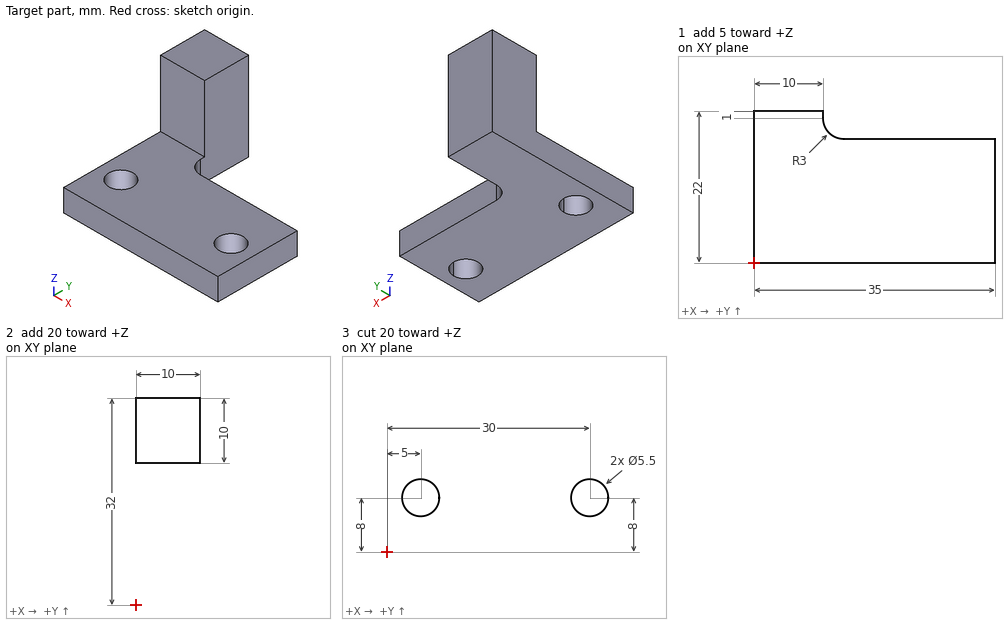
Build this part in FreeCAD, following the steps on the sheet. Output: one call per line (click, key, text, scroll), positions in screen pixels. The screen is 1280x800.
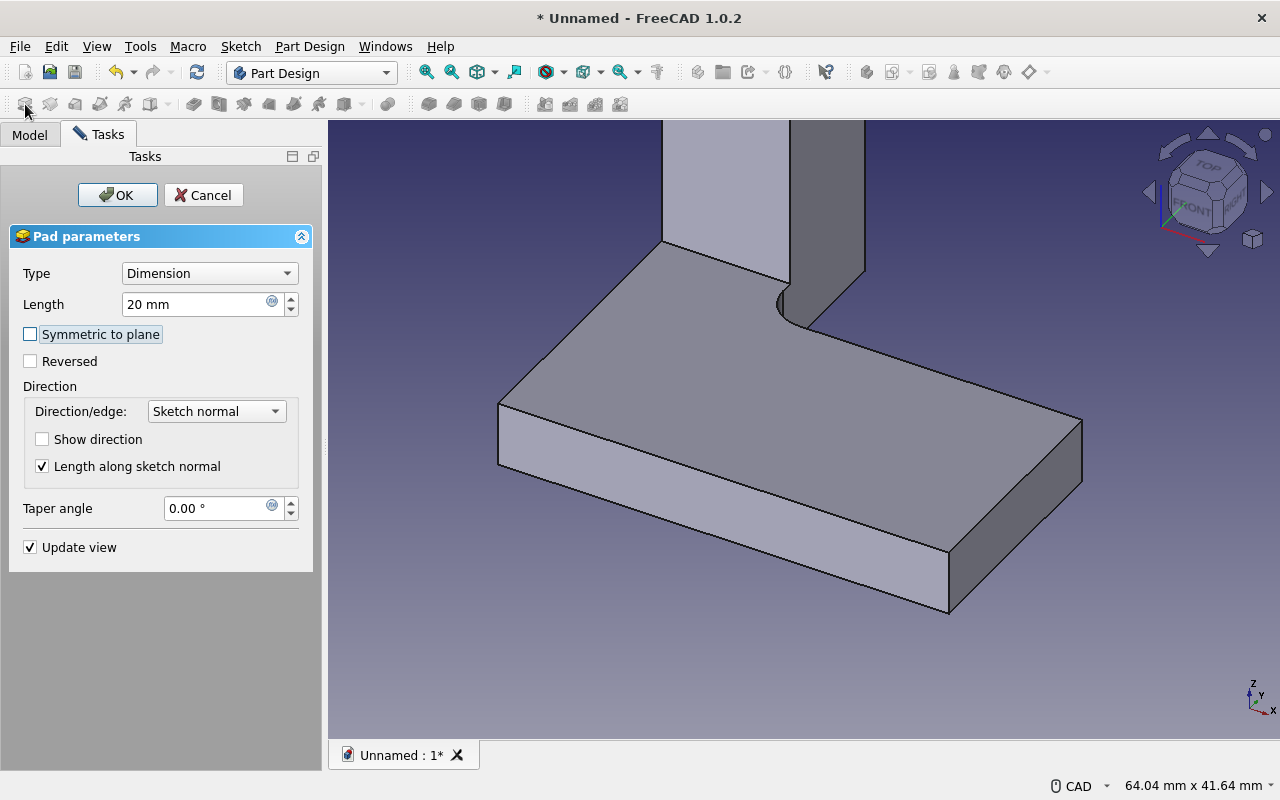
click(118, 195)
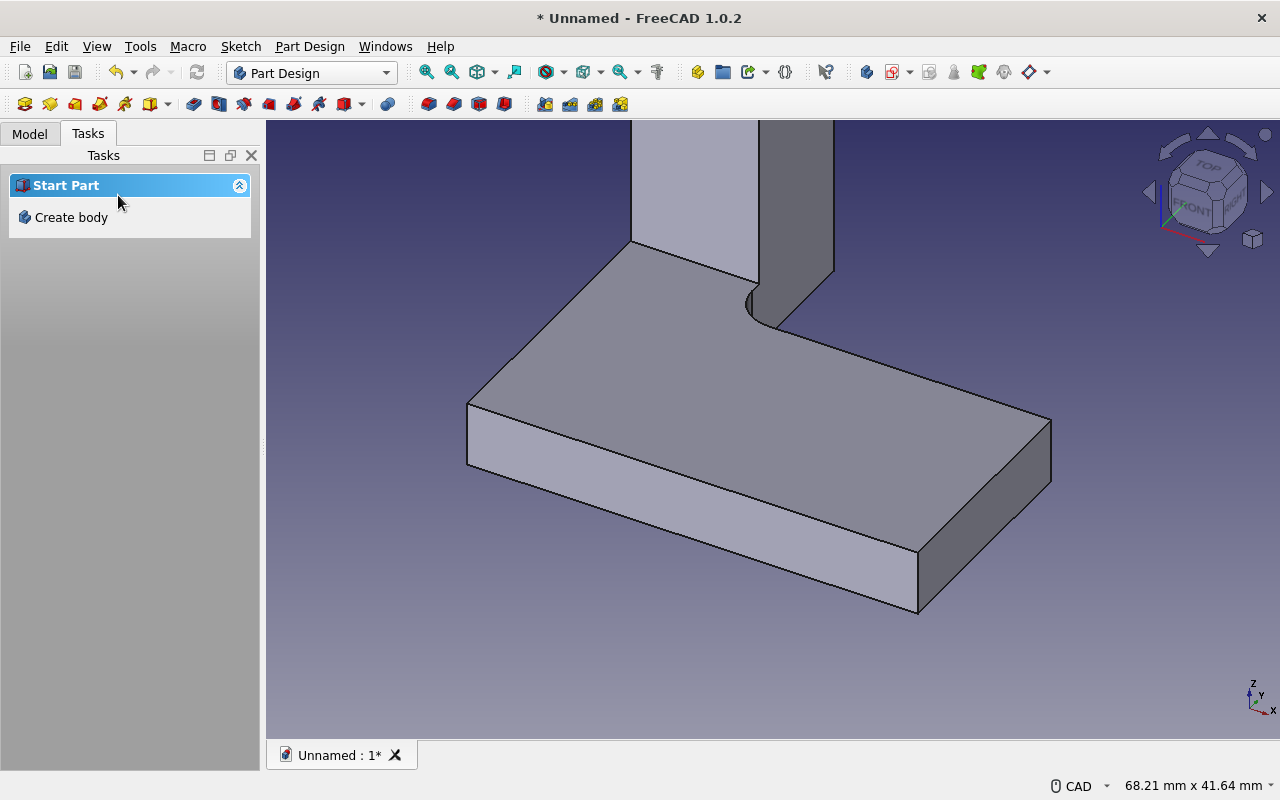
click(427, 72)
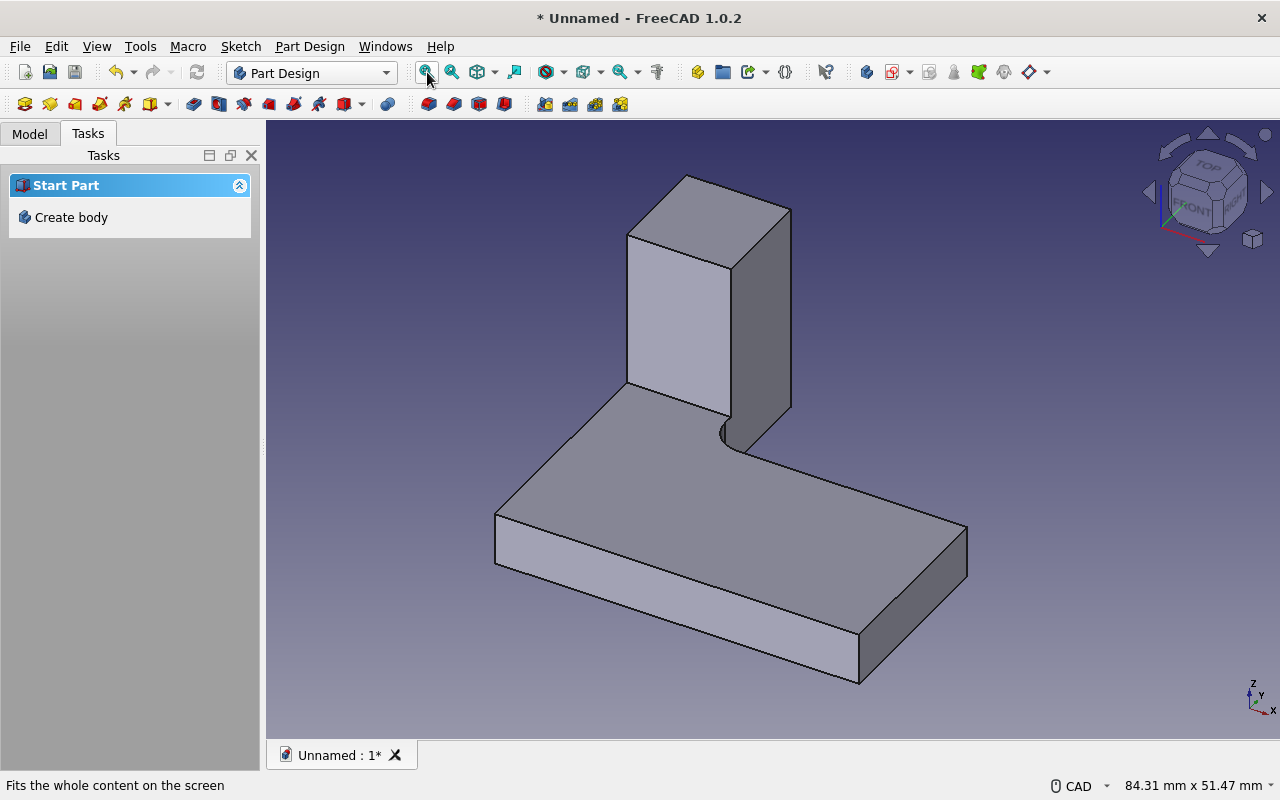
click(892, 72)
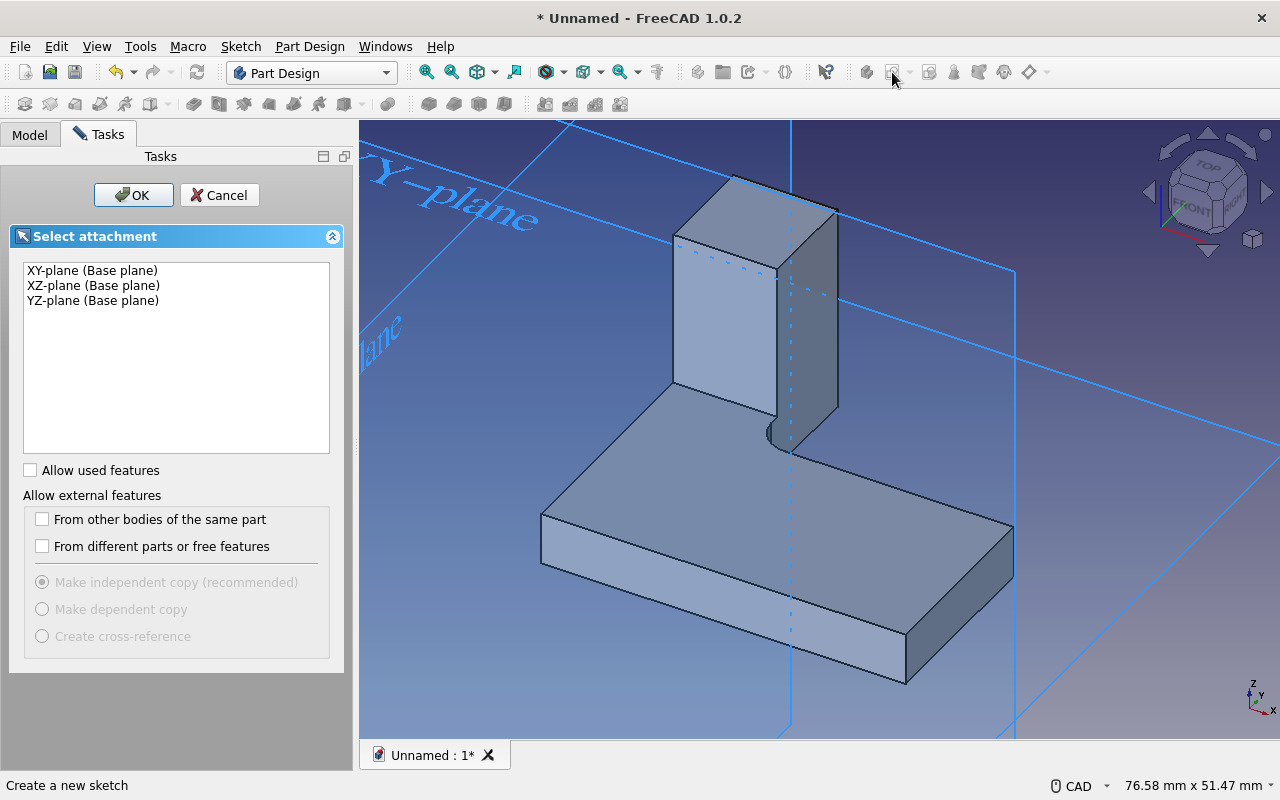
click(84, 270)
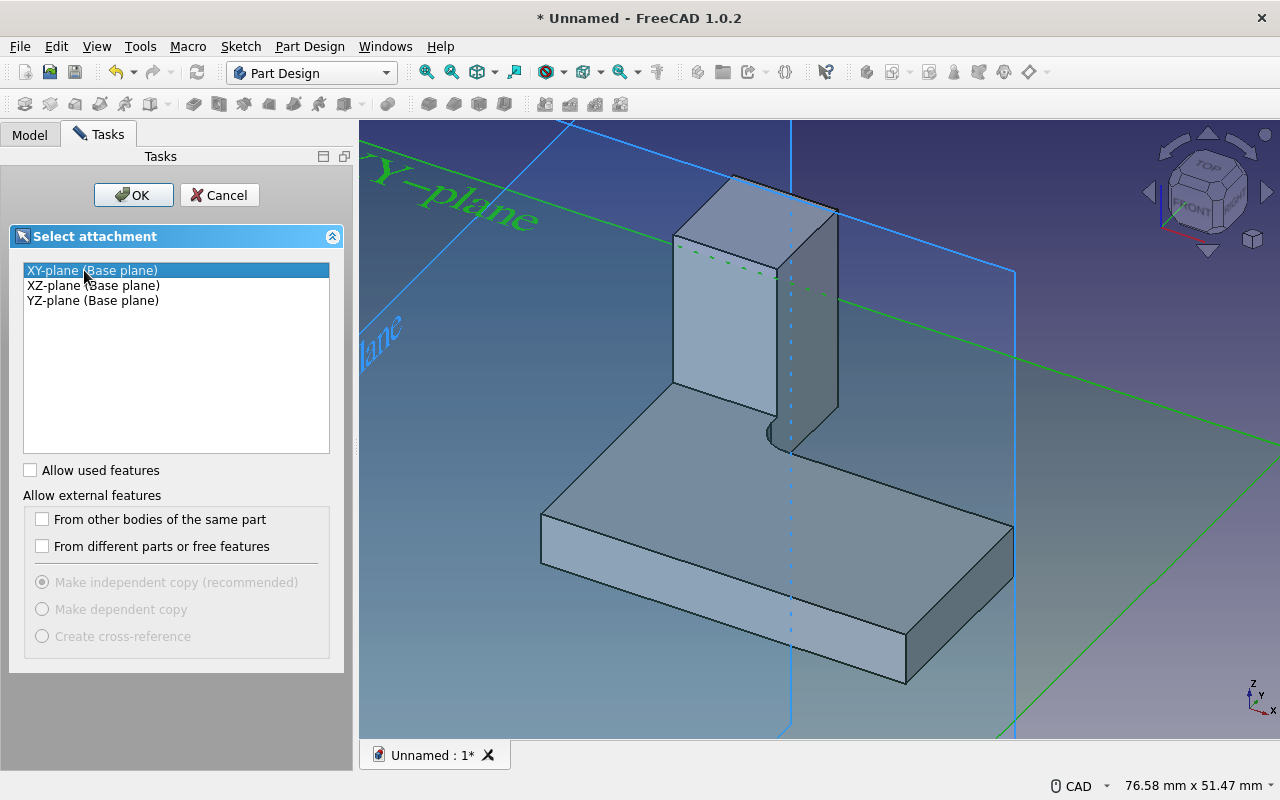
click(134, 195)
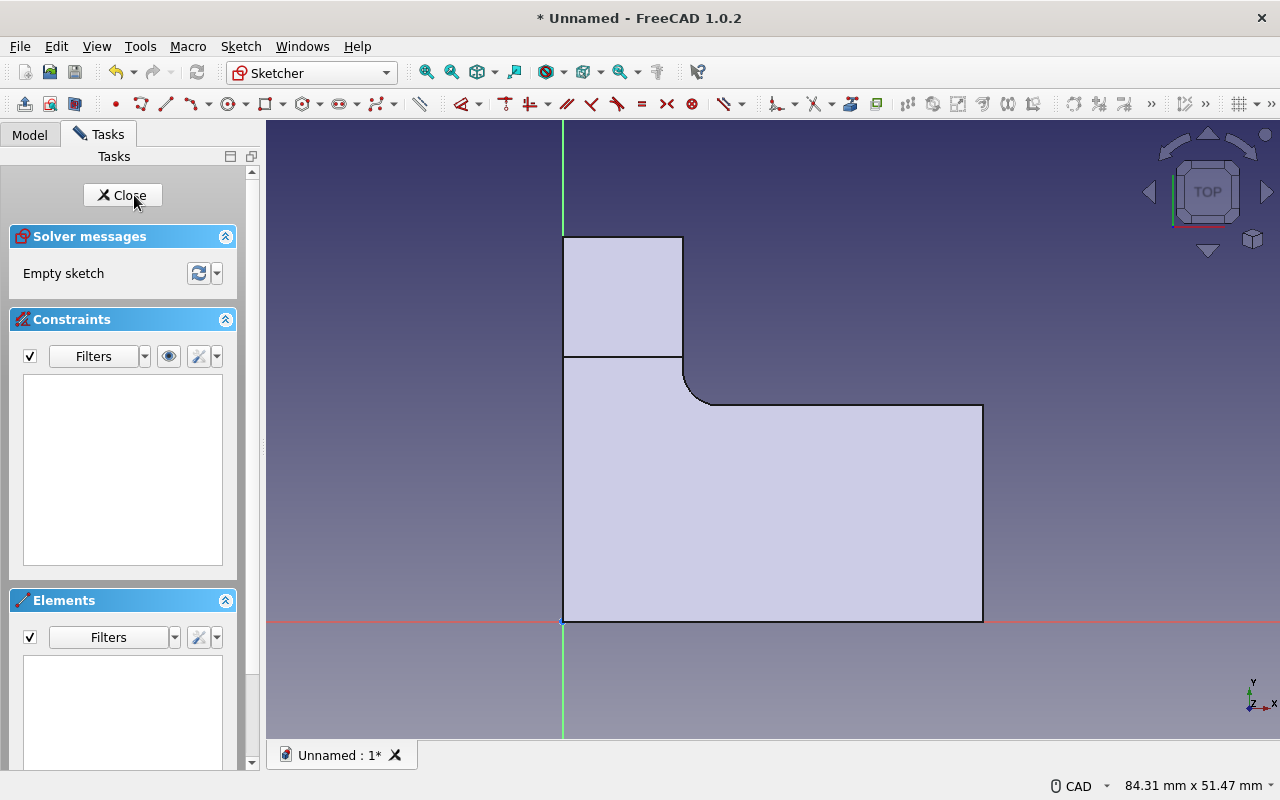
click(75, 104)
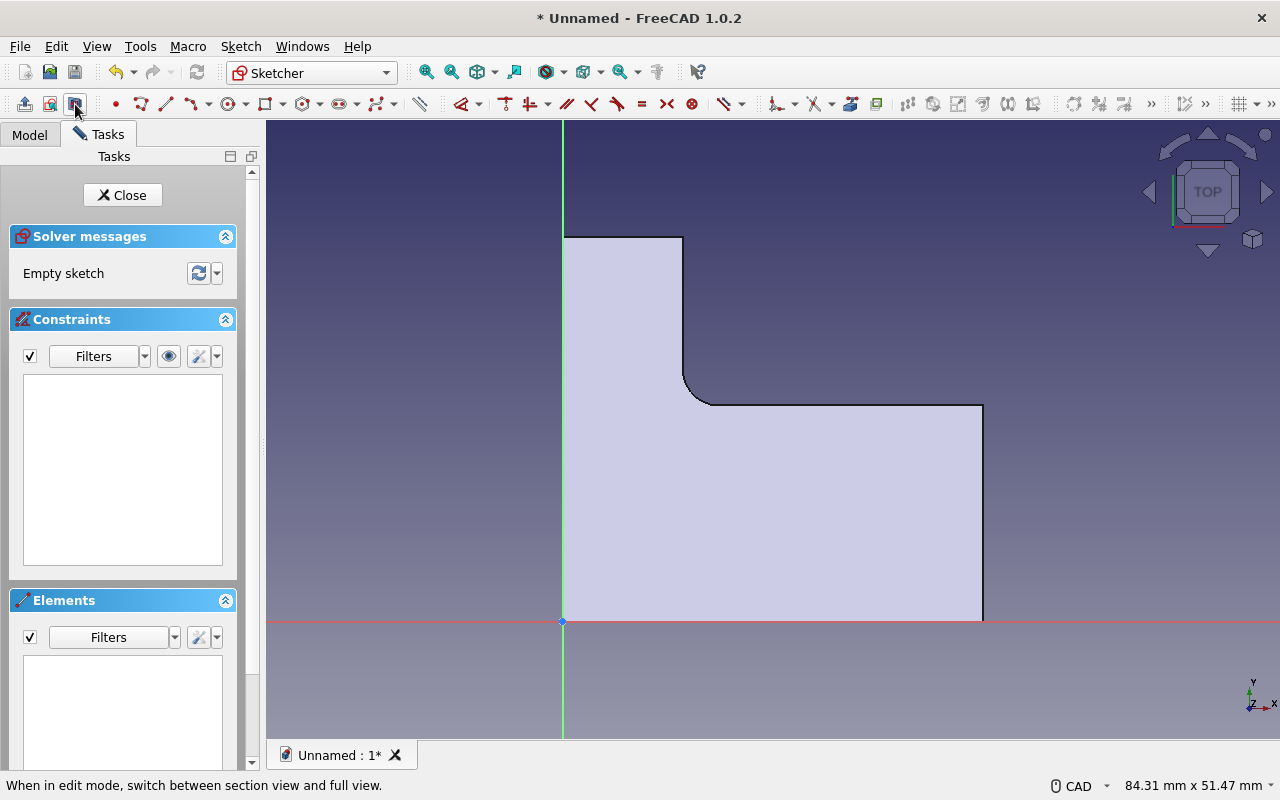
scroll(871, 711, up, 2)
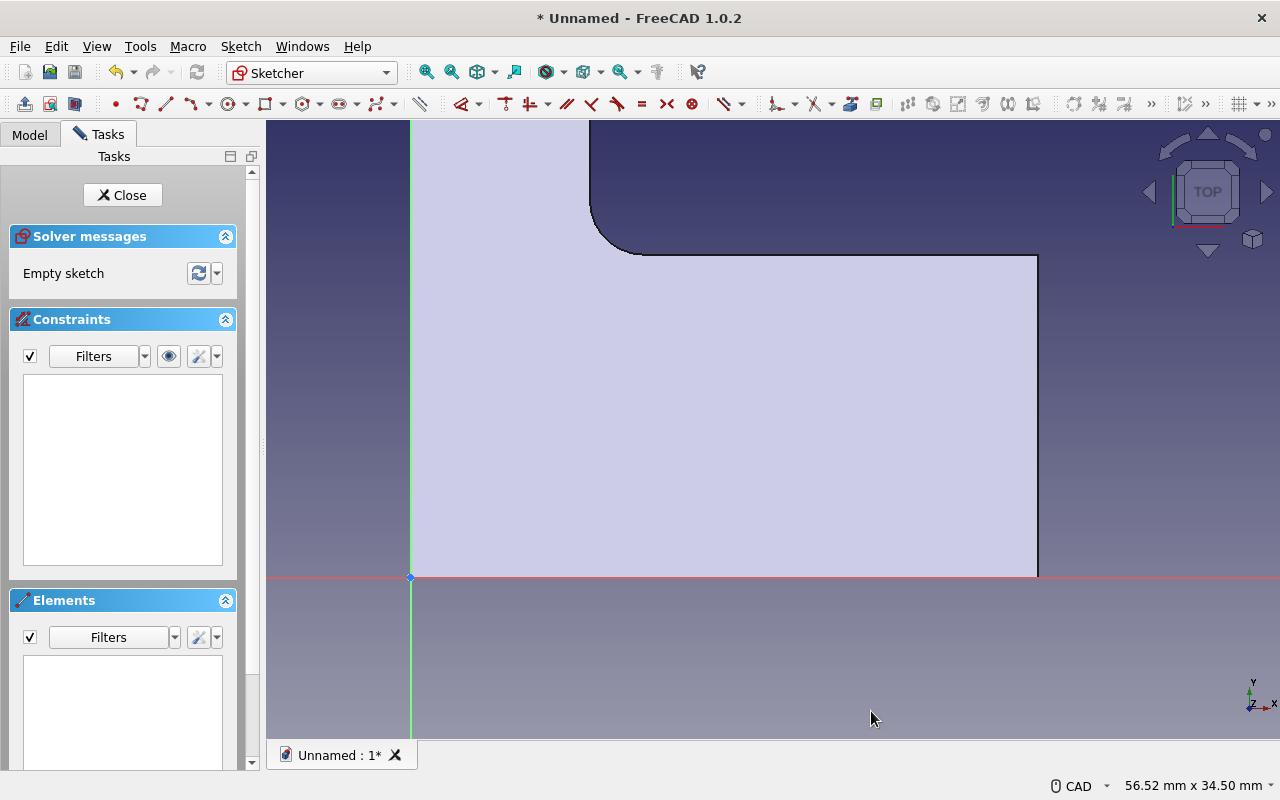
click(228, 104)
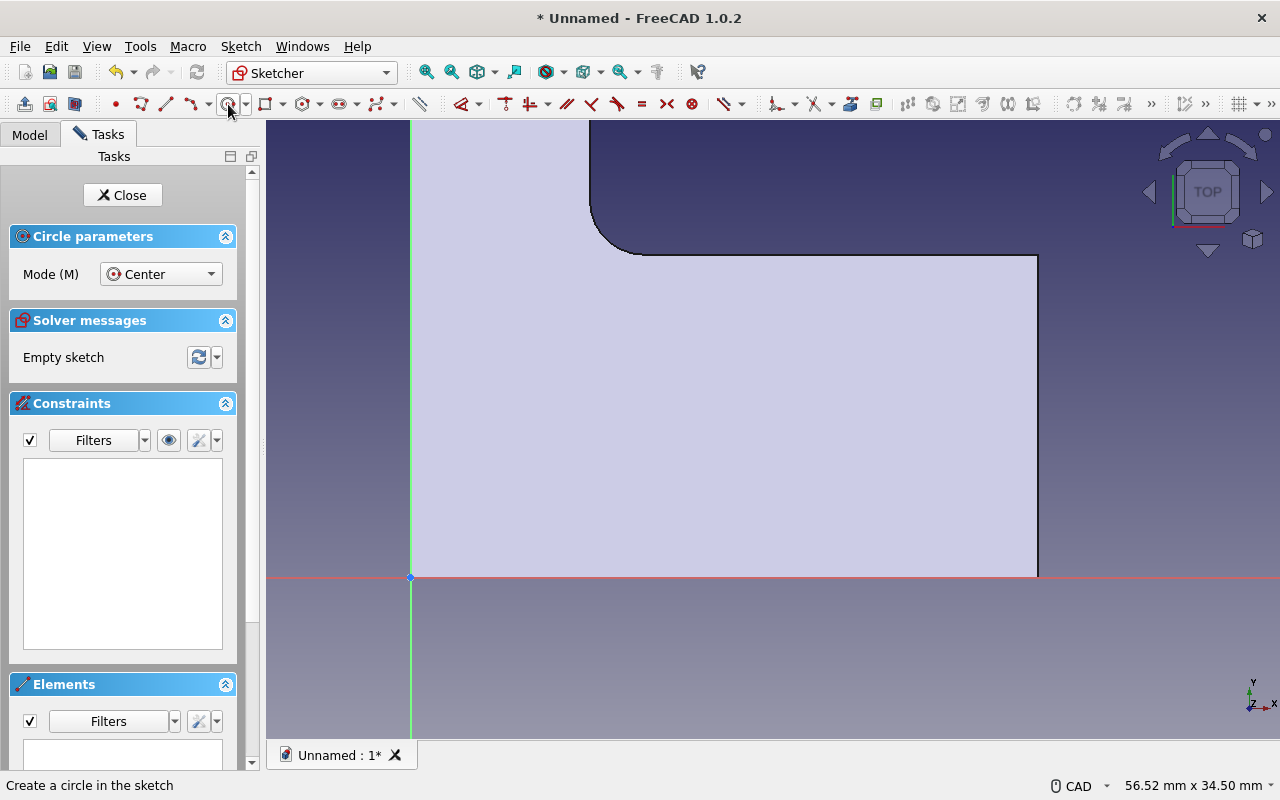
click(949, 434)
move(984, 399)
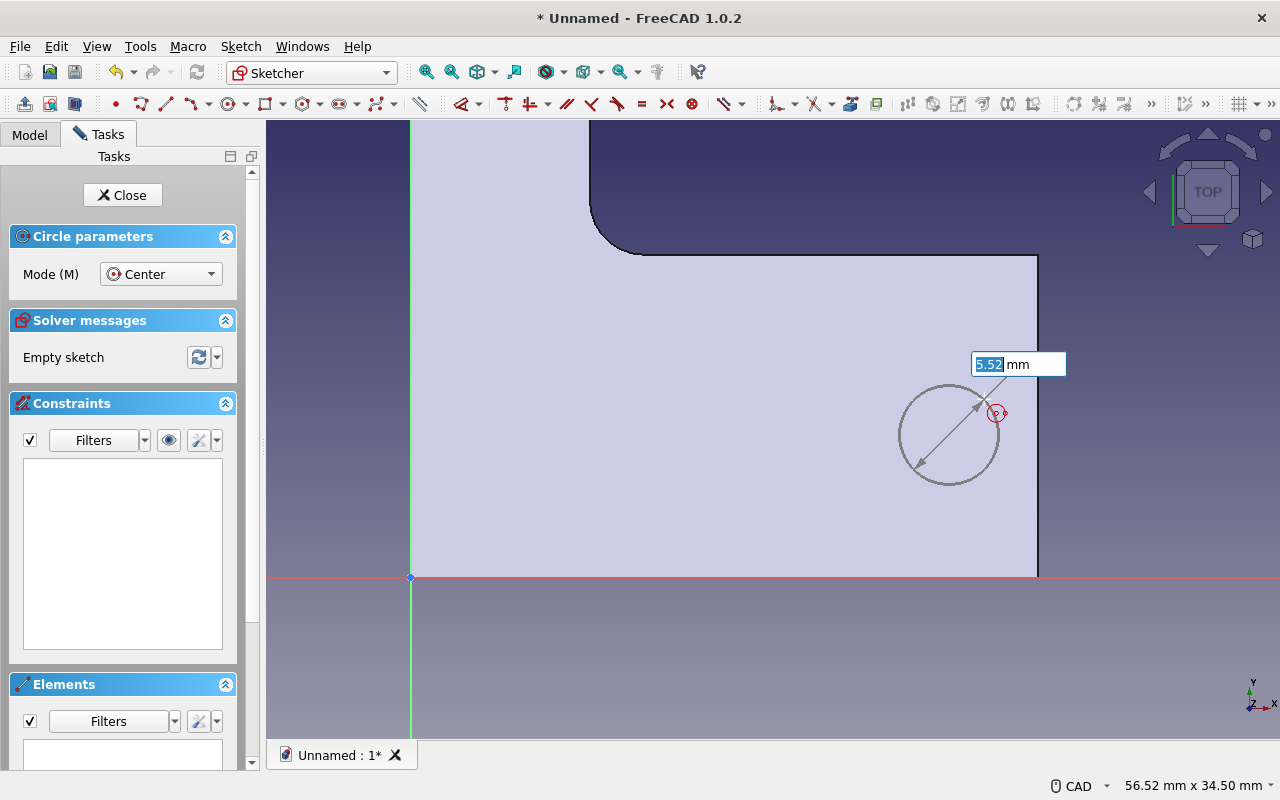
text(5.5)
key(Return)